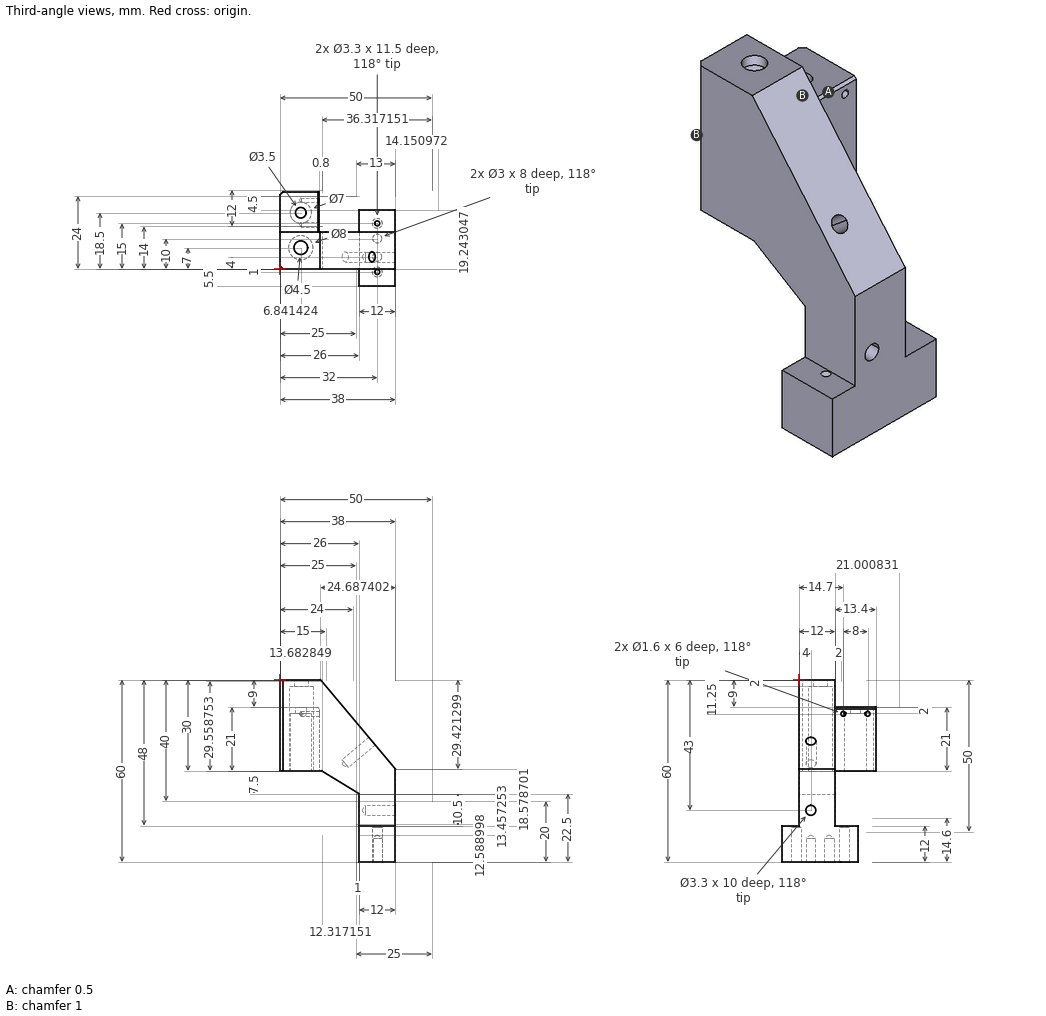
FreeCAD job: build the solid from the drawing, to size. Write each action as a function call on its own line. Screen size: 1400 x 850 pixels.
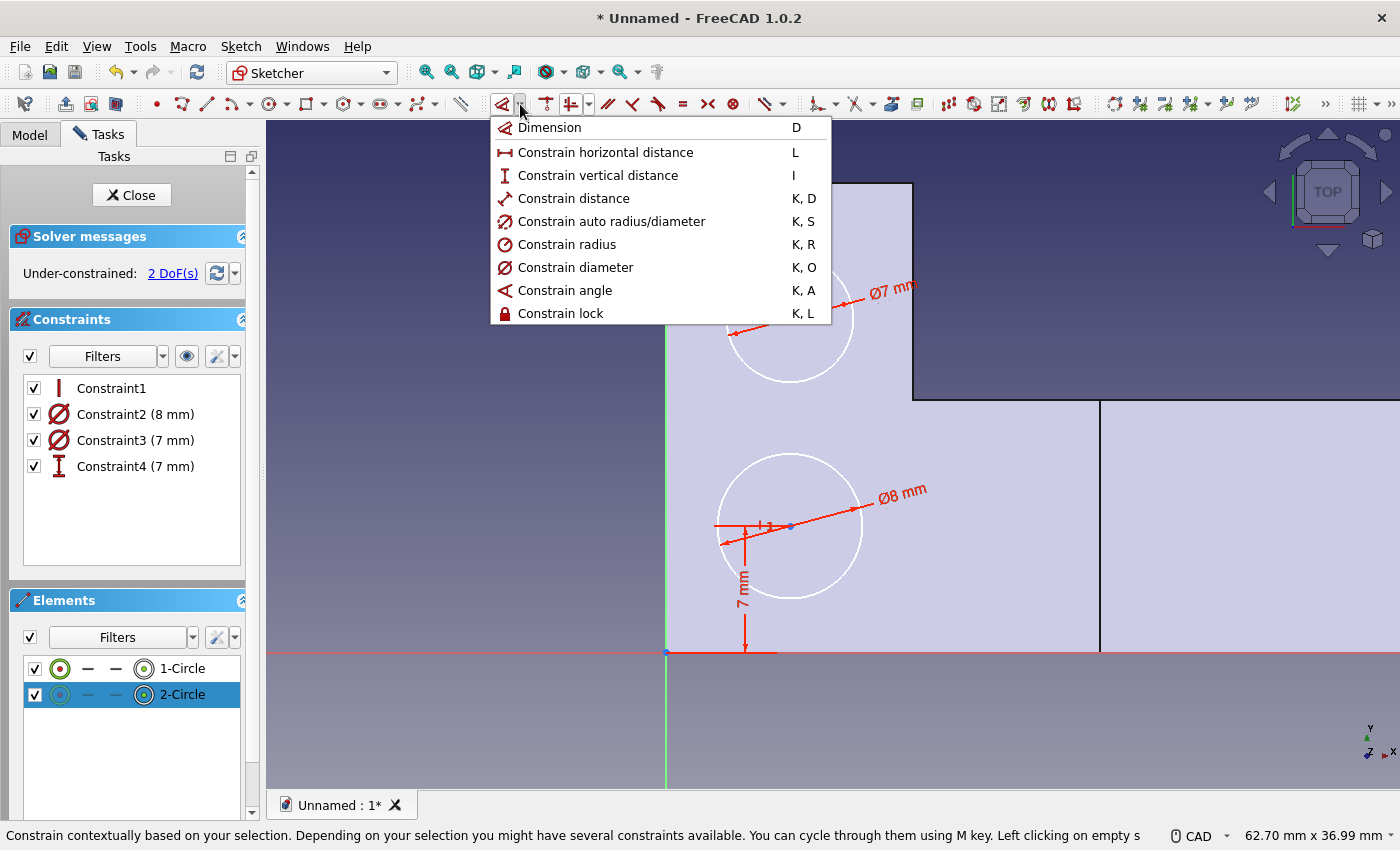
click(661, 176)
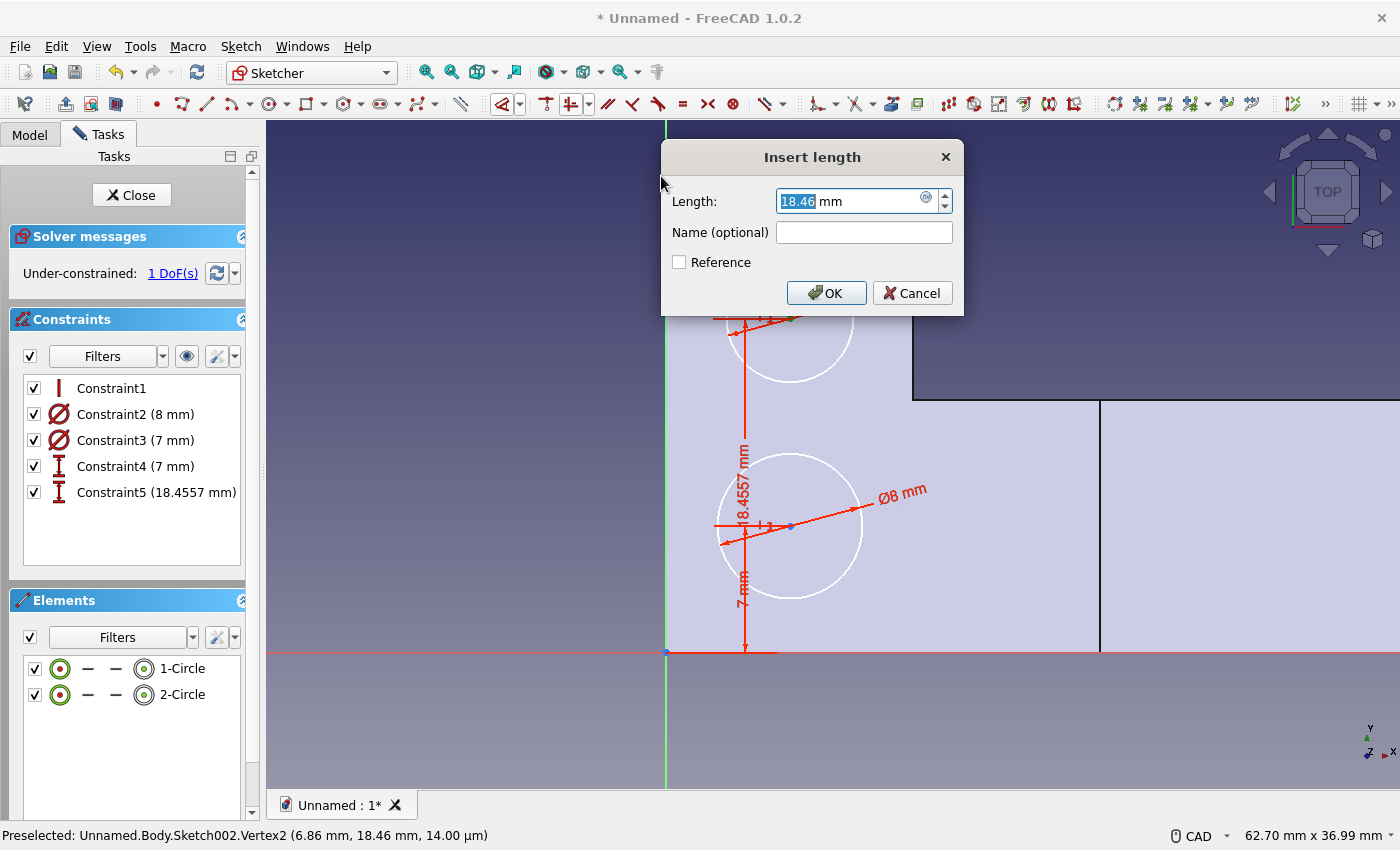
text(18.5)
key(Return)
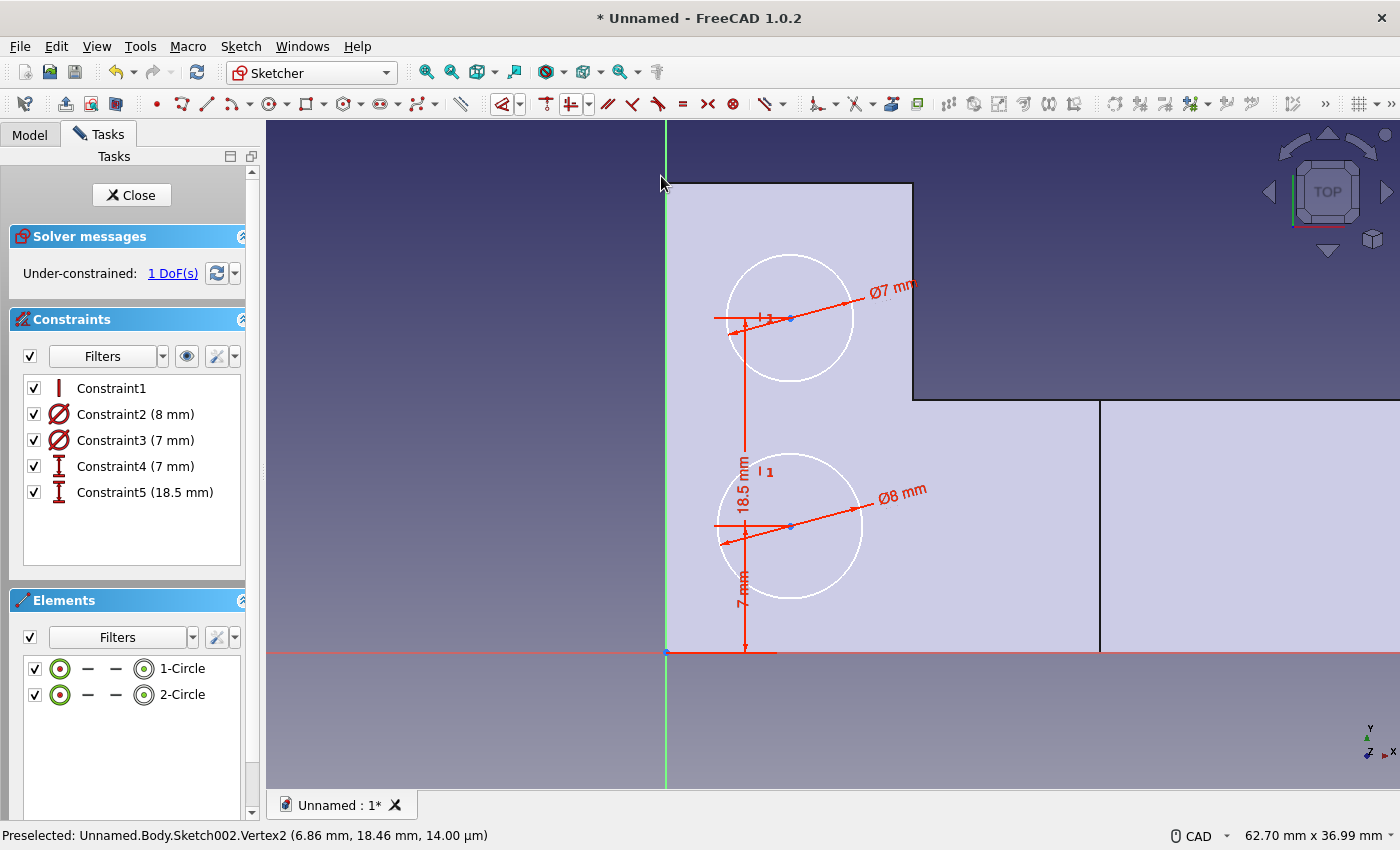
click(790, 526)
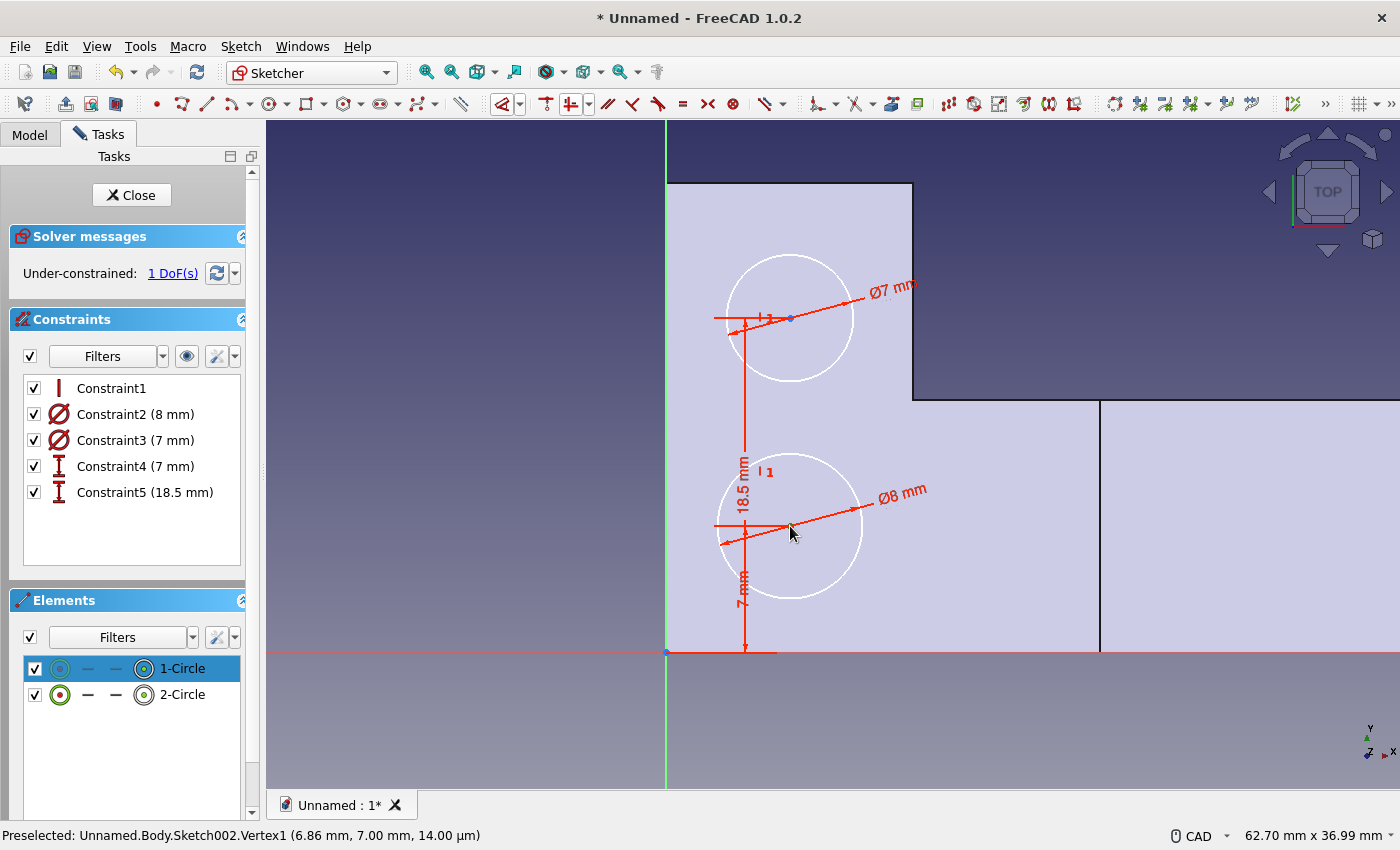
click(520, 104)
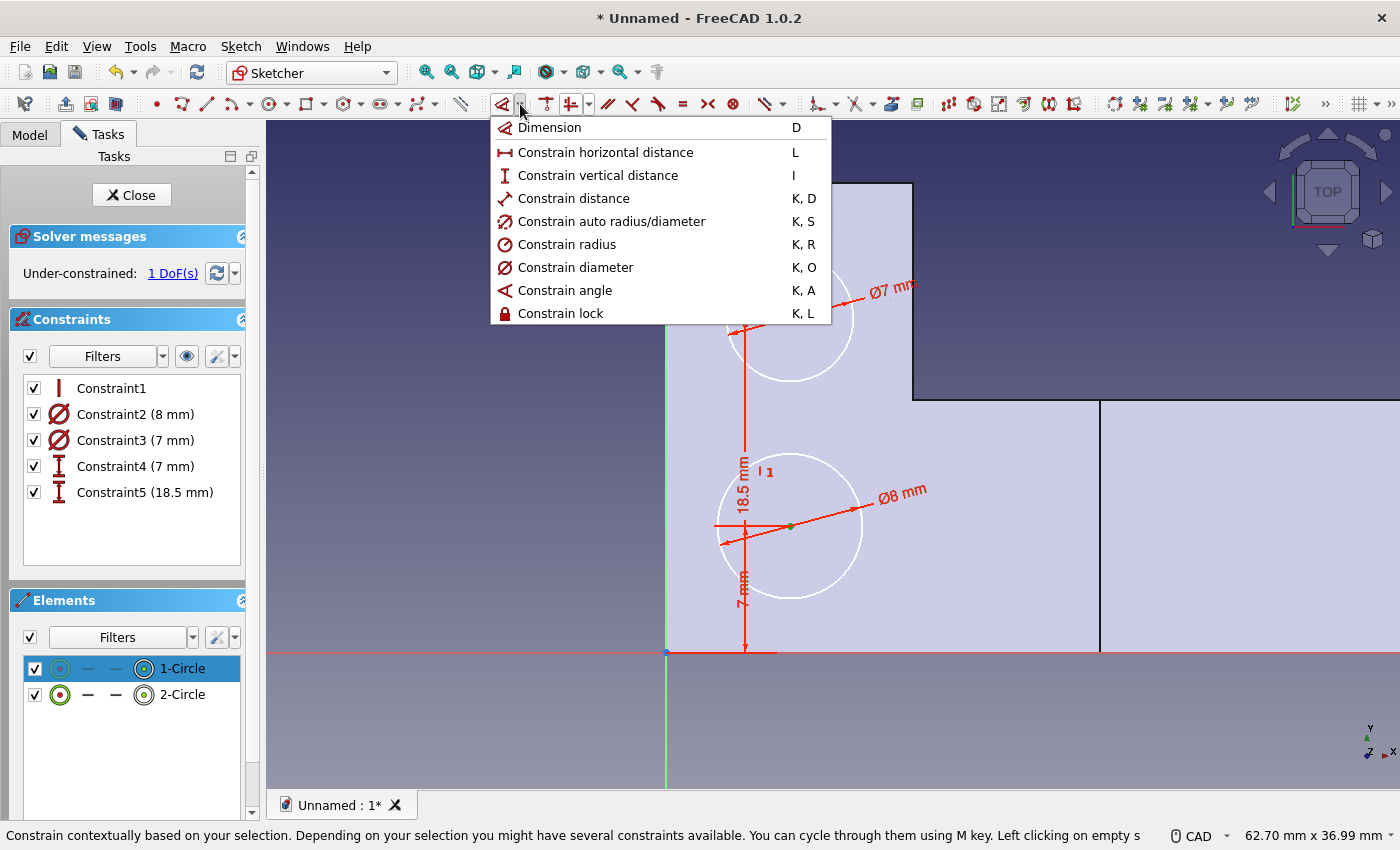
click(661, 152)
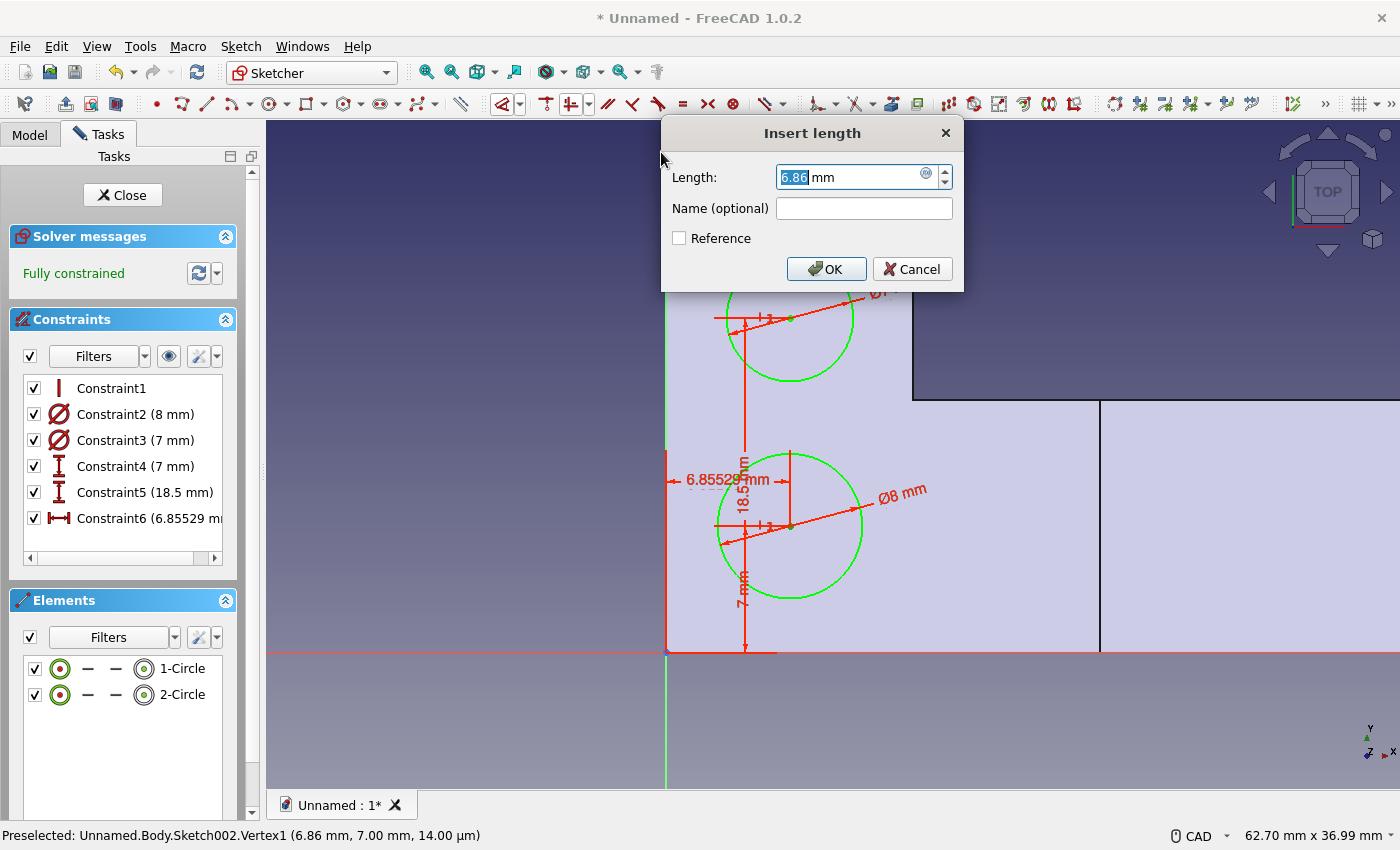
text(6.841424)
key(Return)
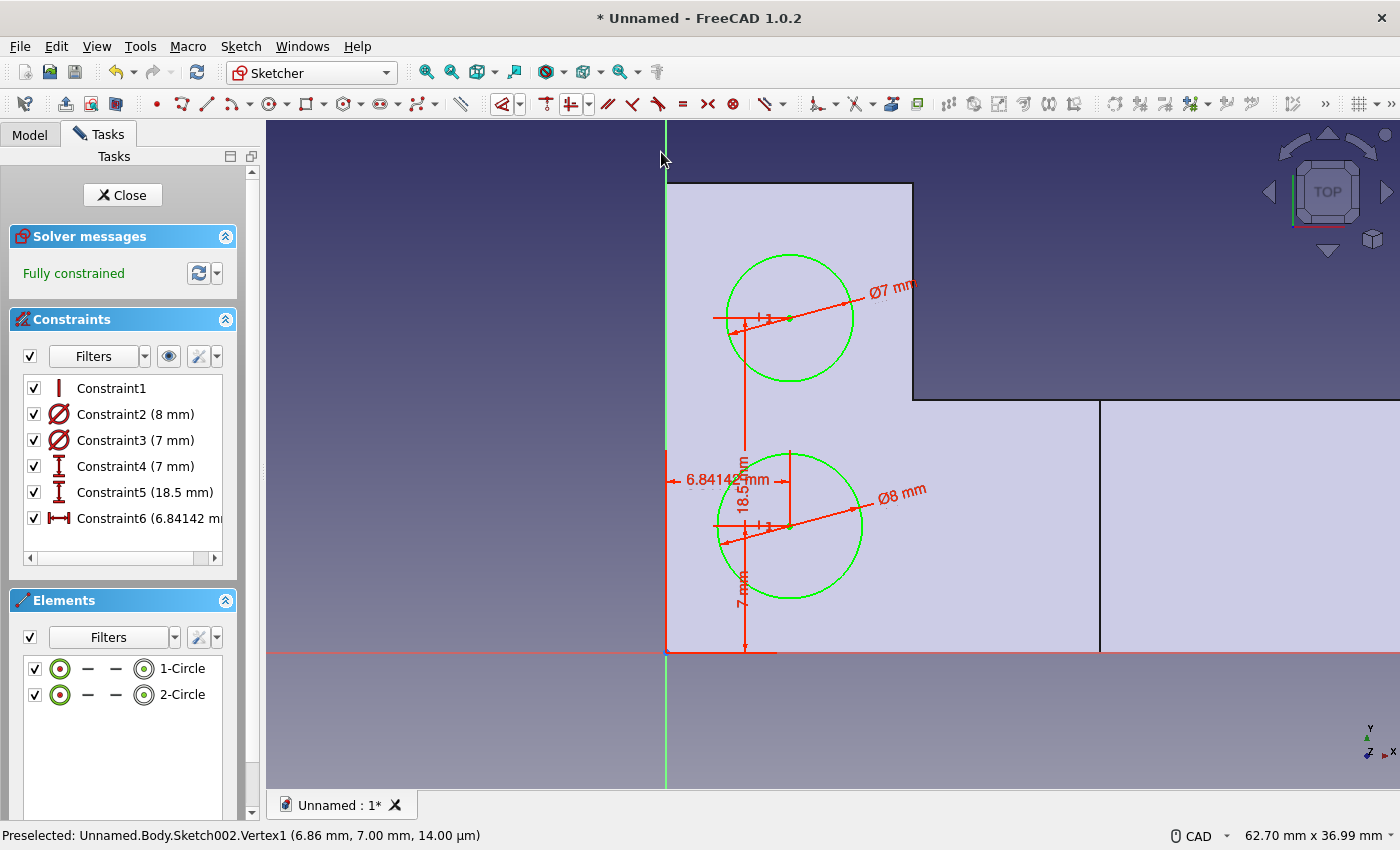
click(123, 195)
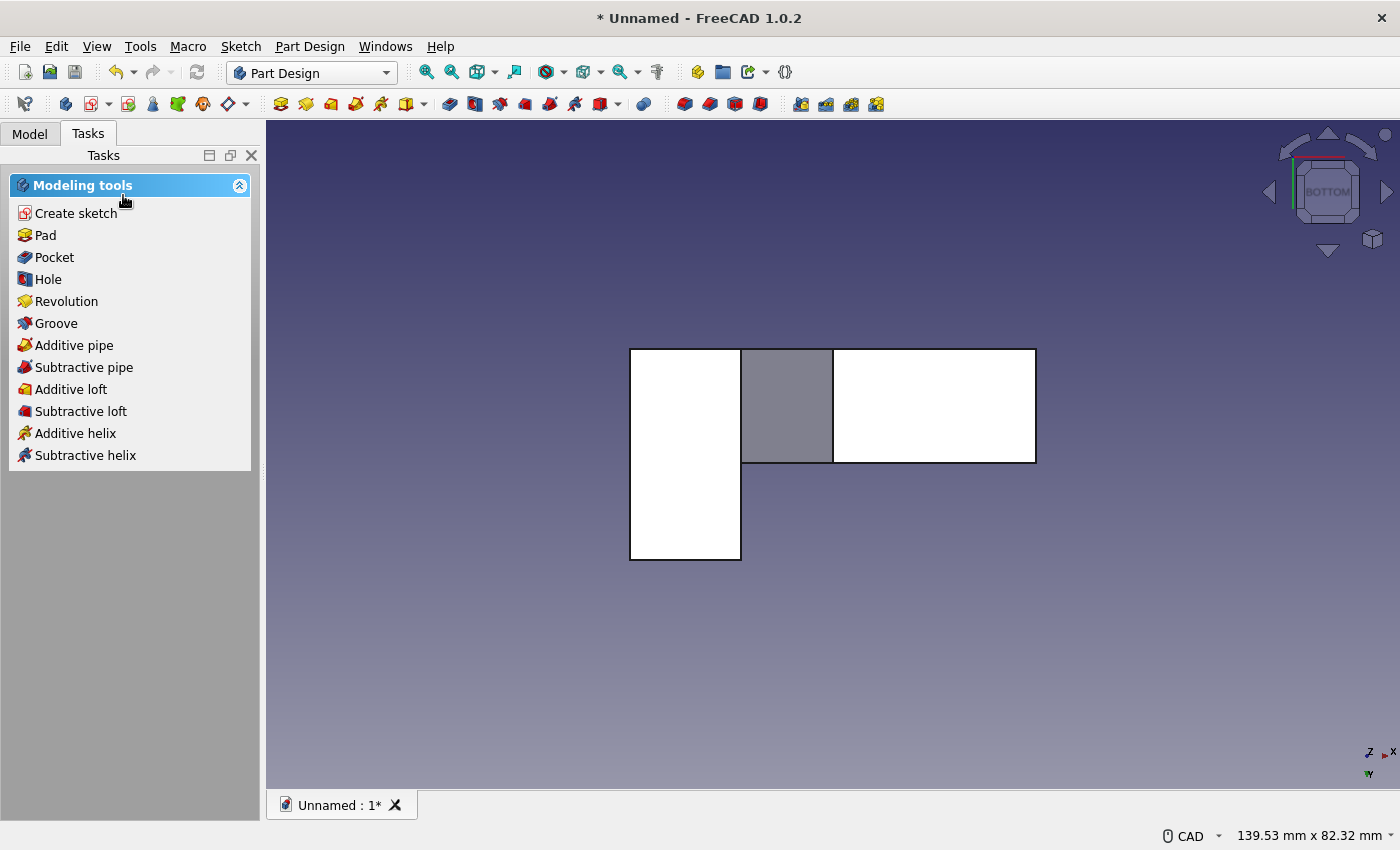
click(450, 104)